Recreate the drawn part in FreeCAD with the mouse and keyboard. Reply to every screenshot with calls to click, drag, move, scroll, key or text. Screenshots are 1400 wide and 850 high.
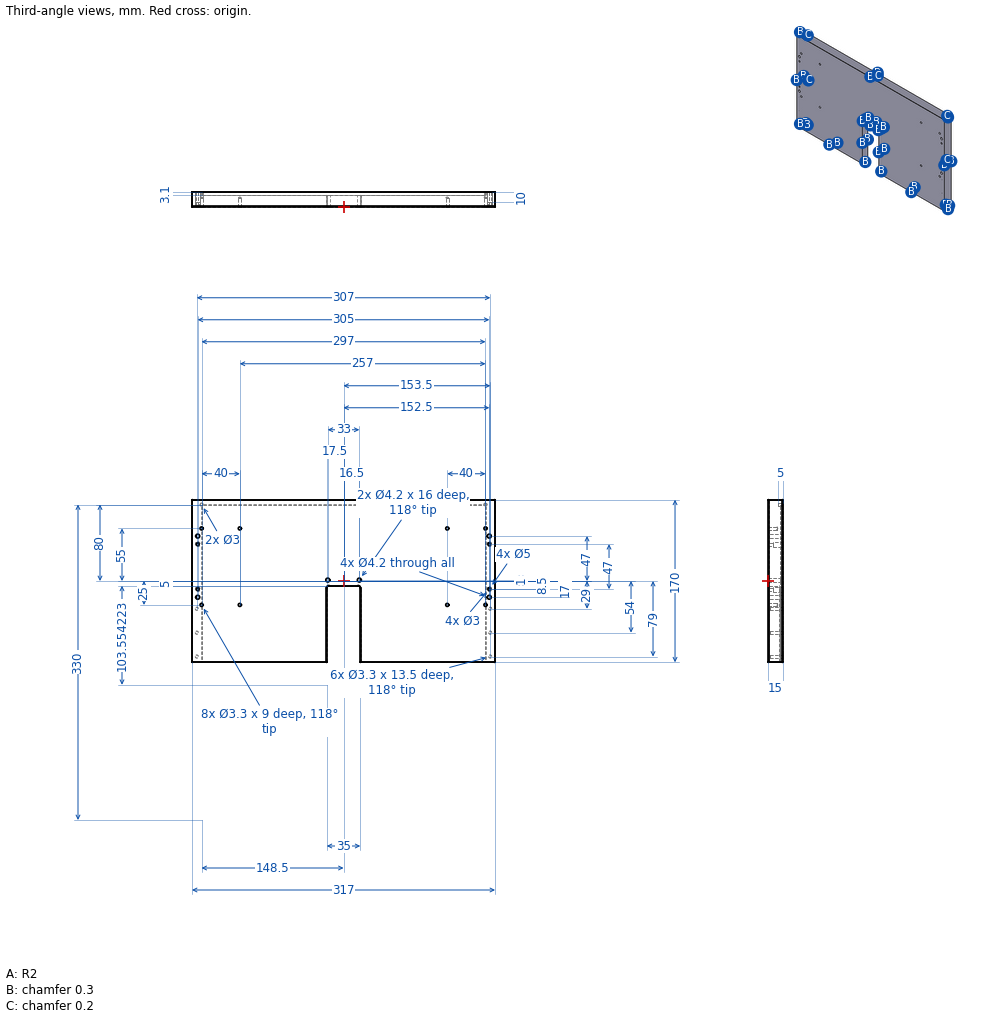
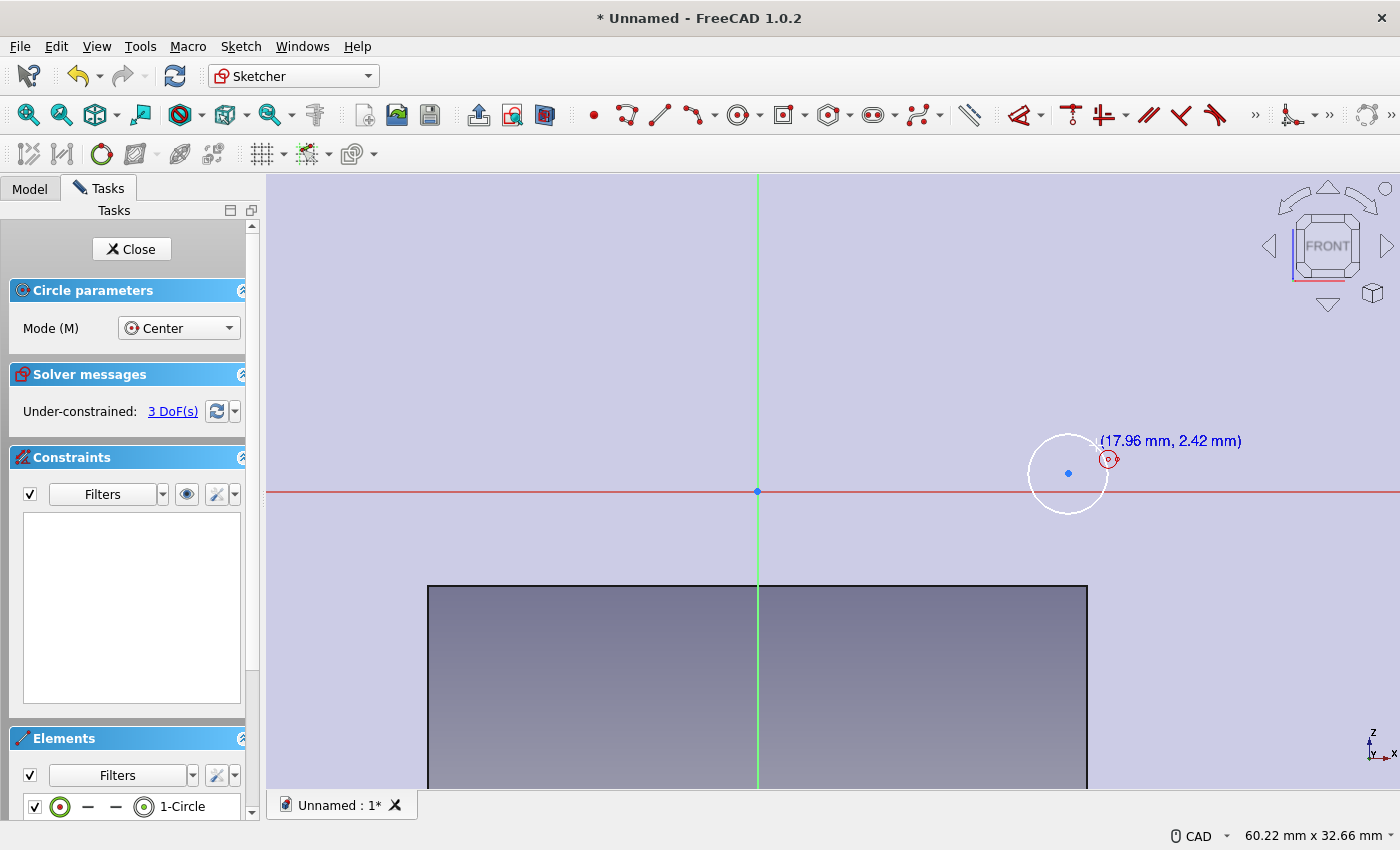
click(447, 473)
click(475, 445)
key(Escape)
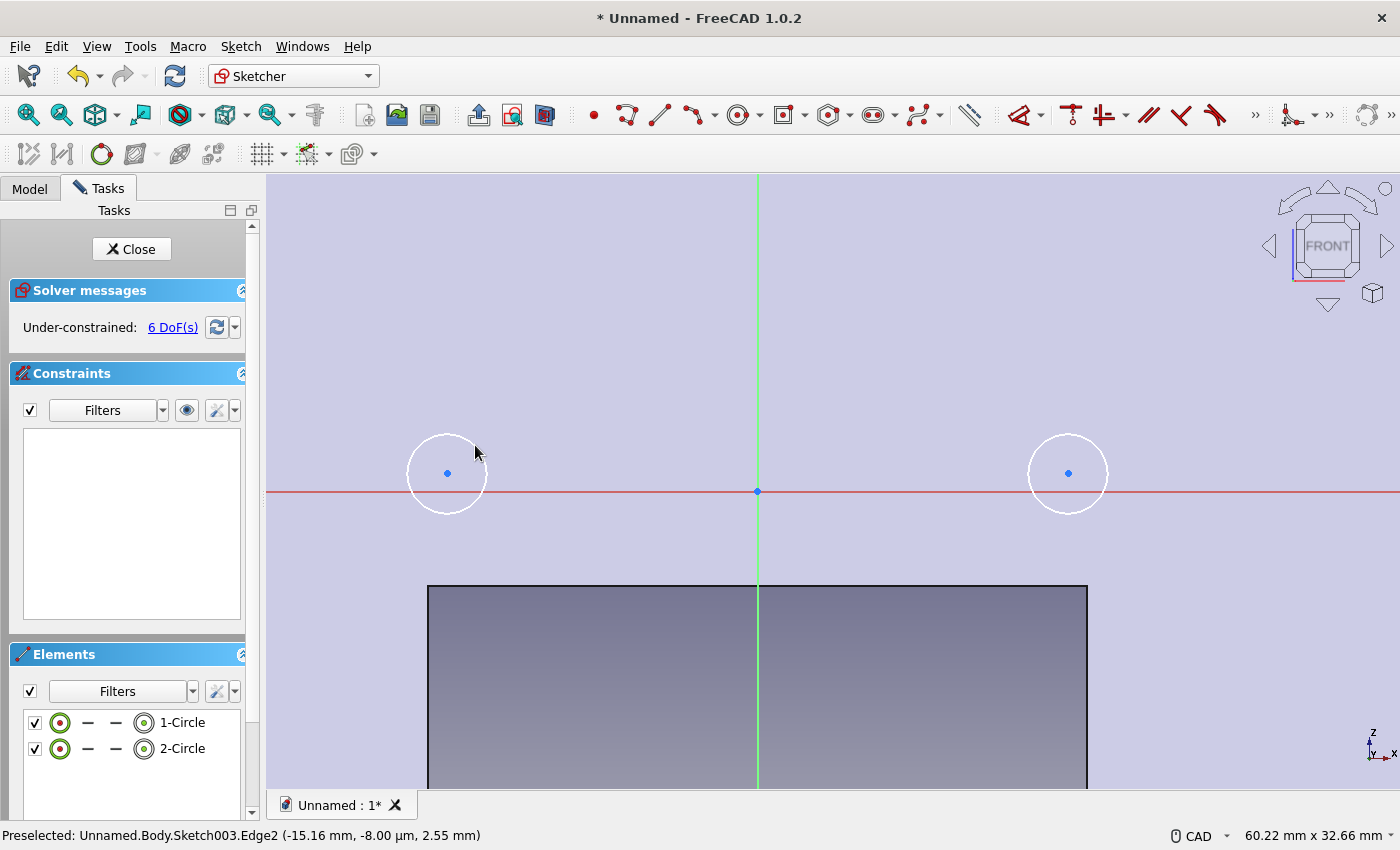
click(1096, 446)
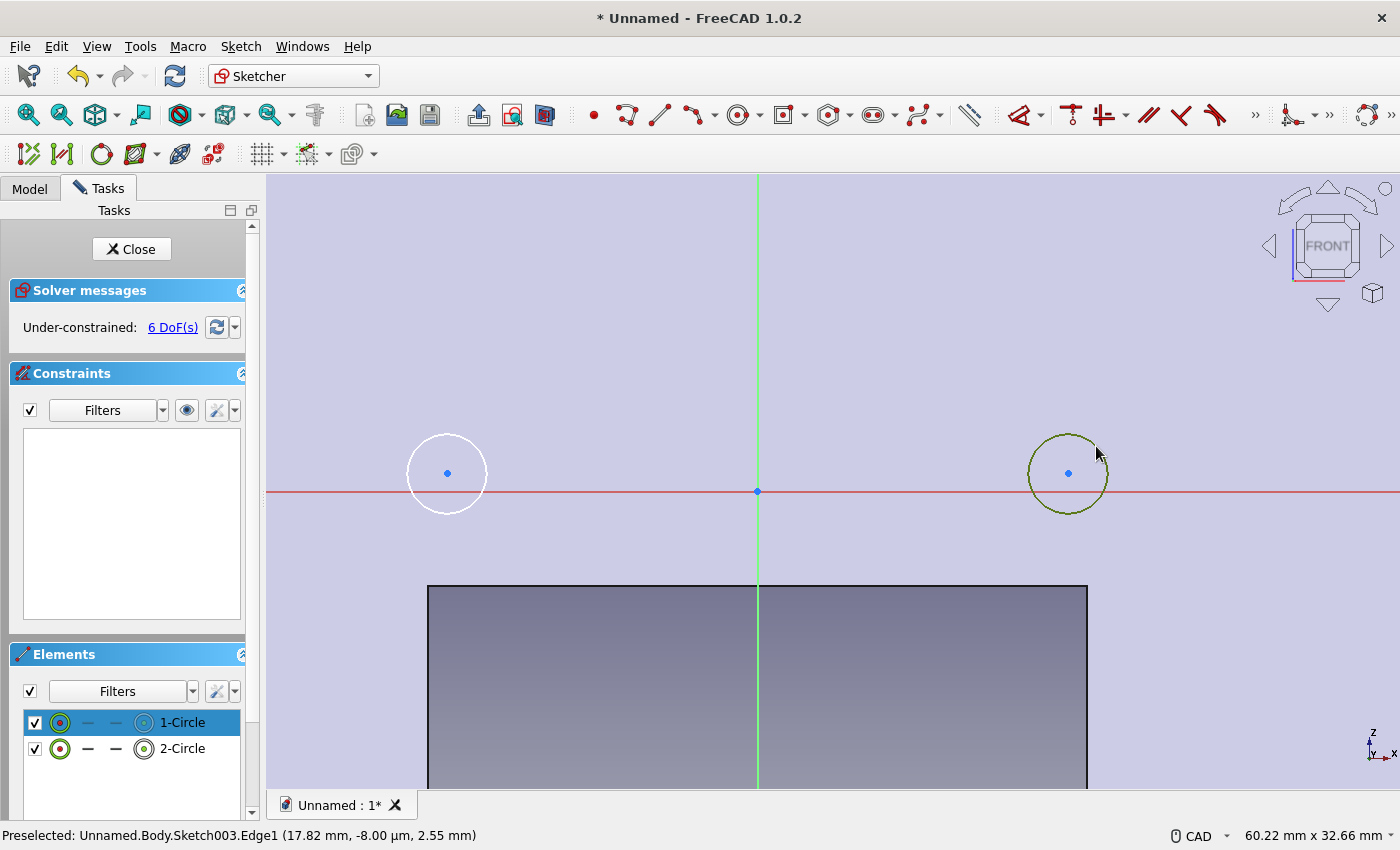
click(475, 446)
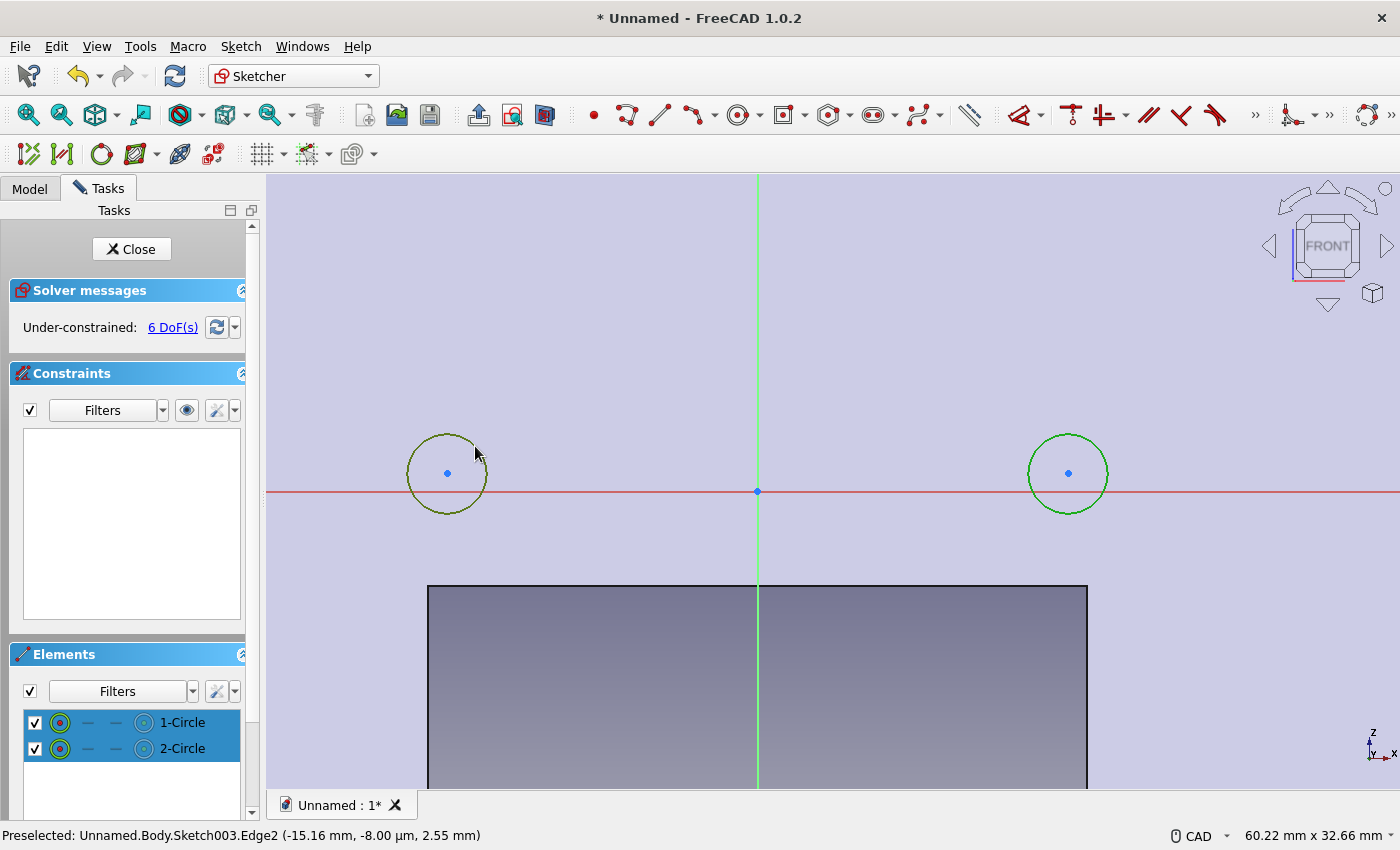
key(e)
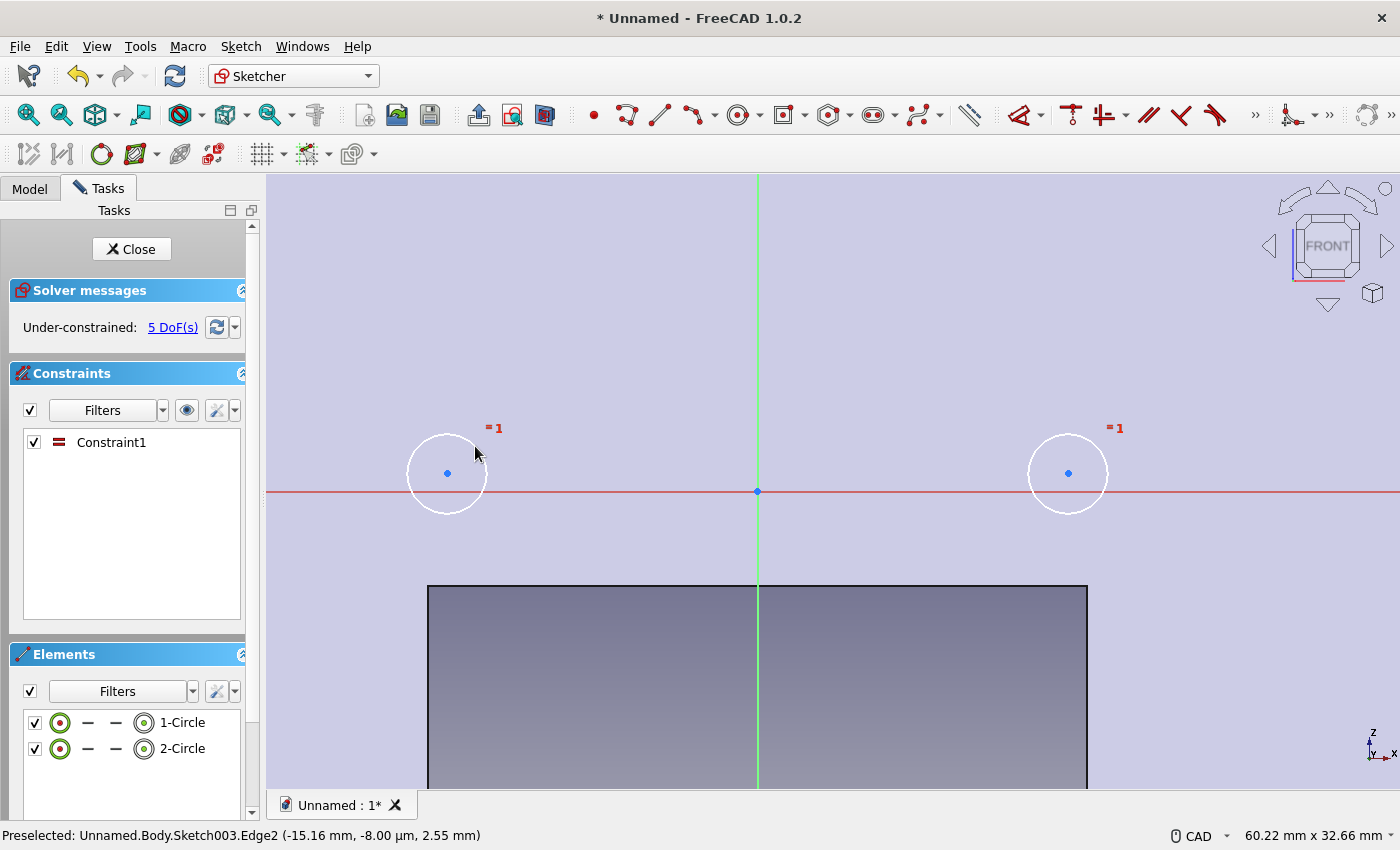
click(1068, 474)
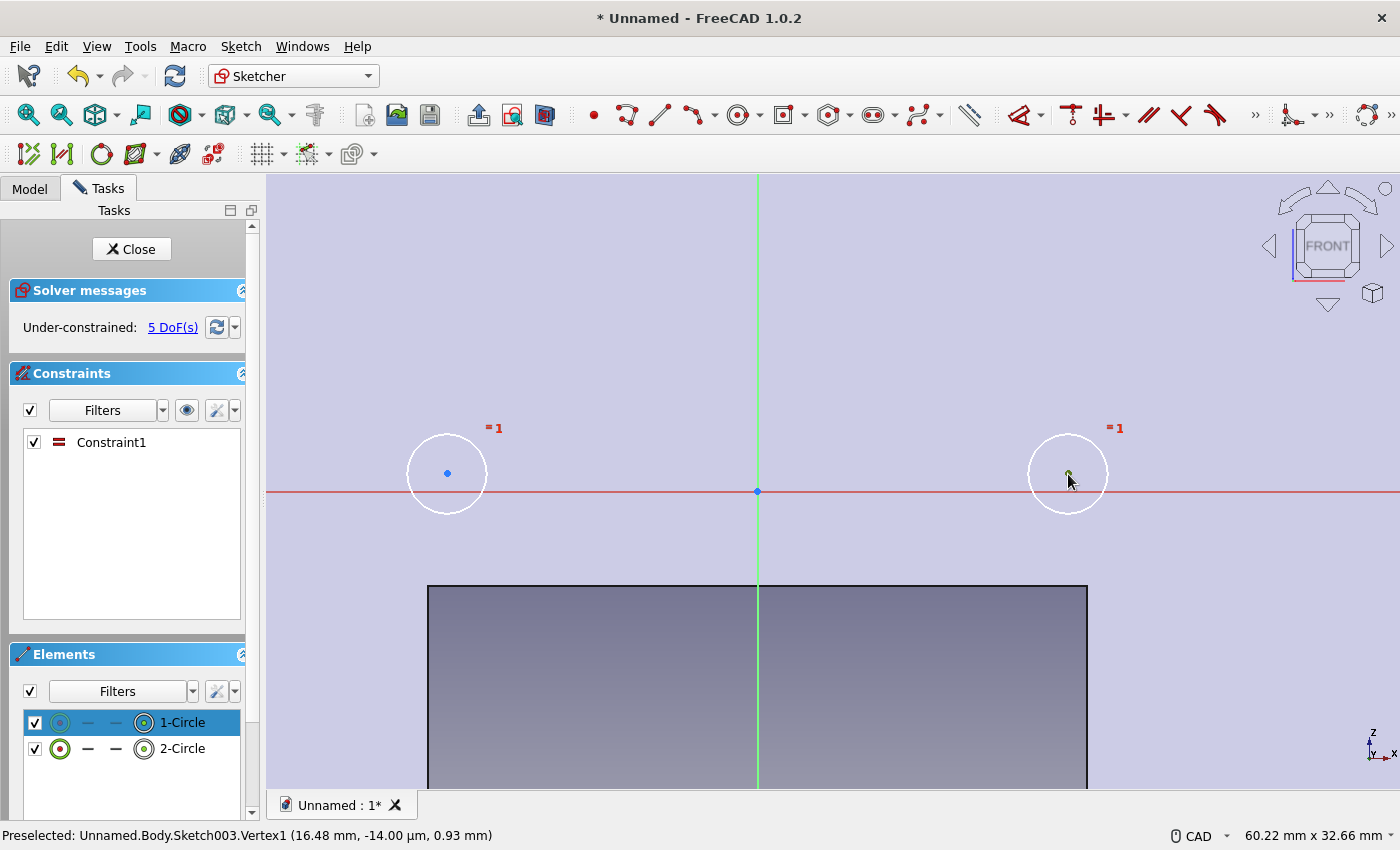
click(447, 474)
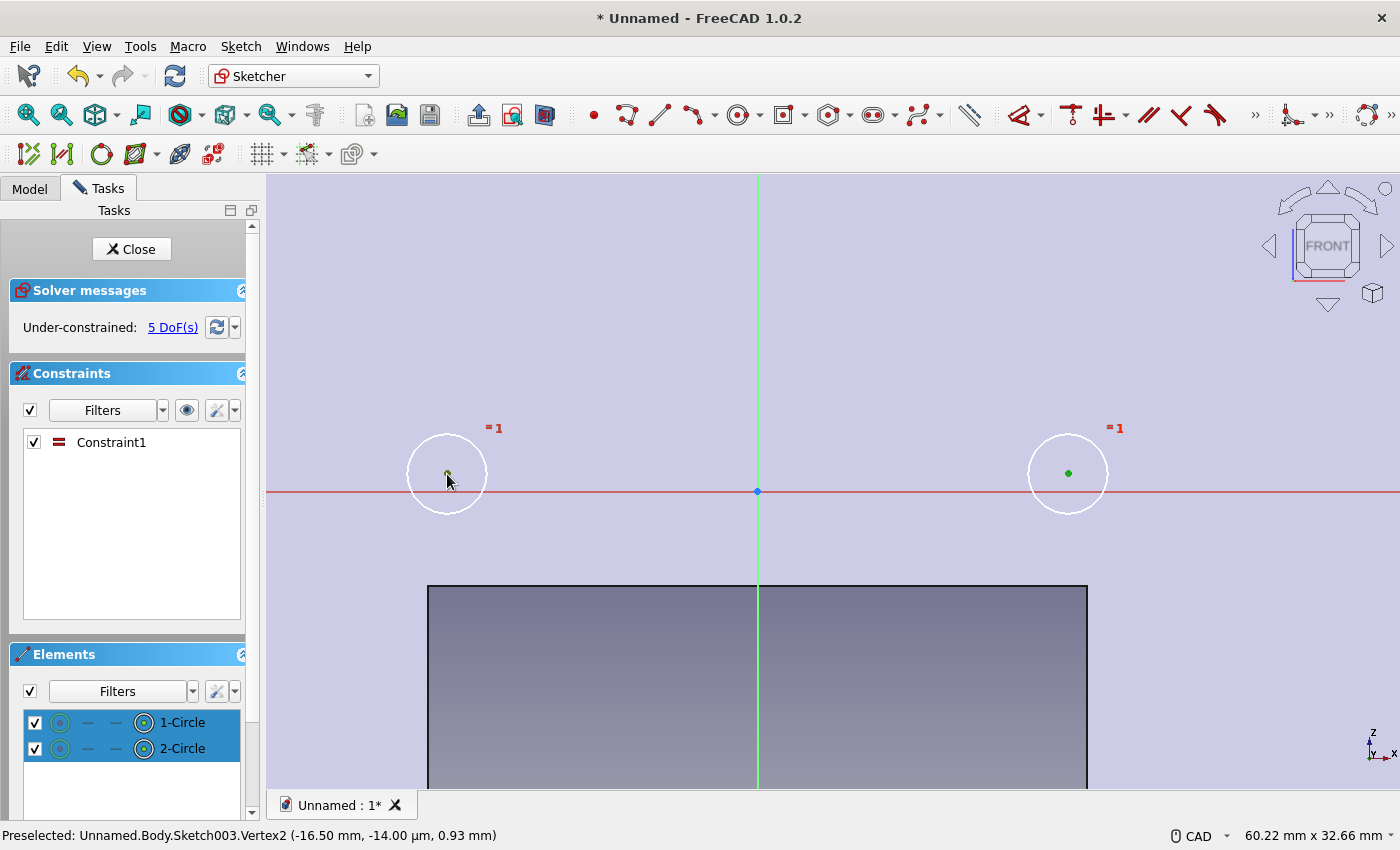
key(h)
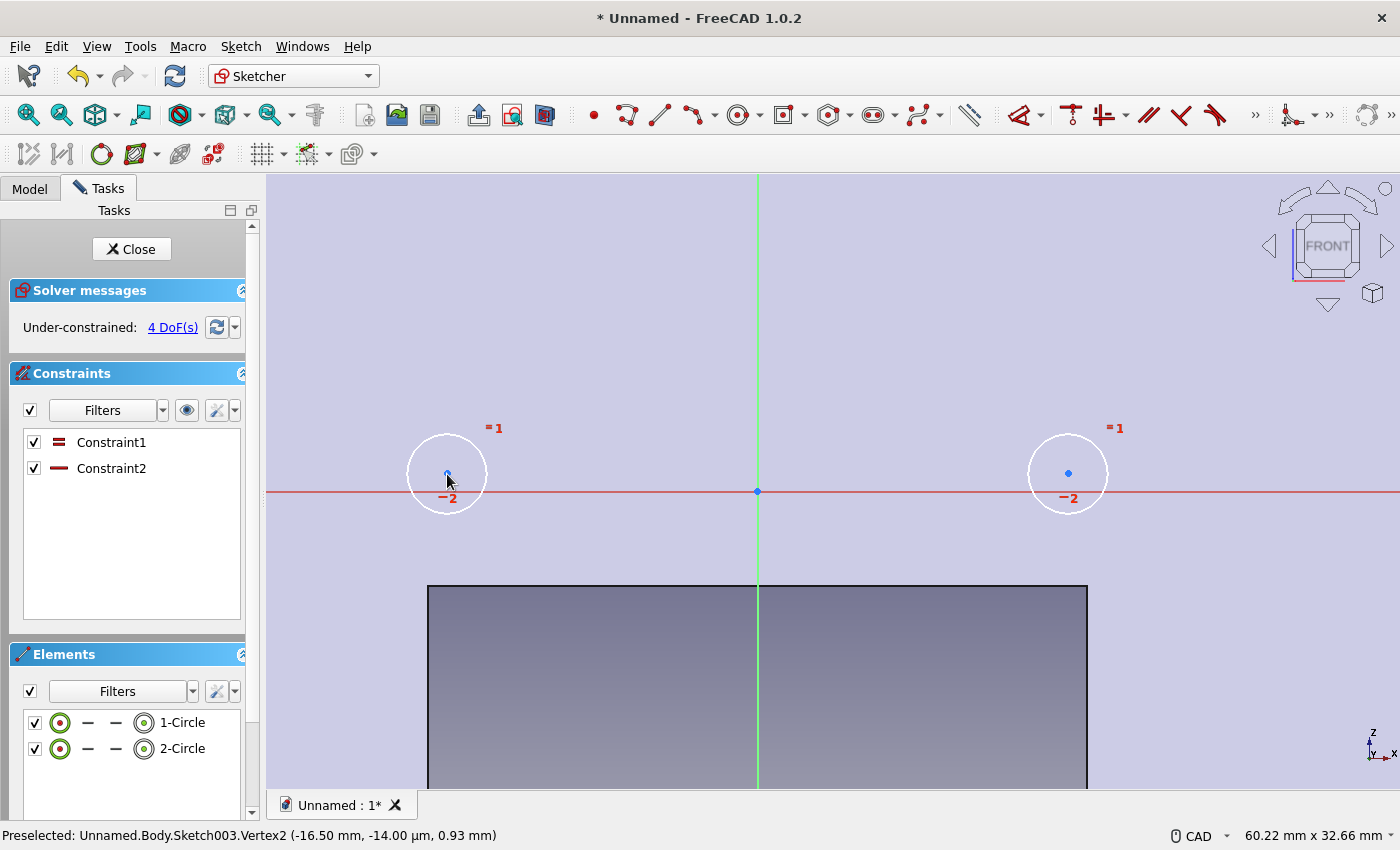
click(1018, 116)